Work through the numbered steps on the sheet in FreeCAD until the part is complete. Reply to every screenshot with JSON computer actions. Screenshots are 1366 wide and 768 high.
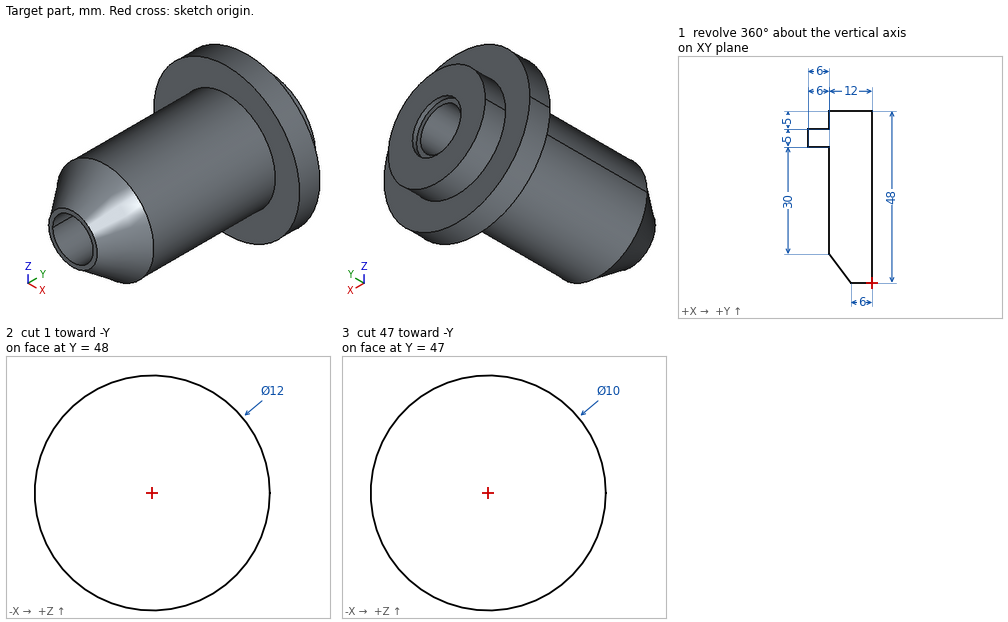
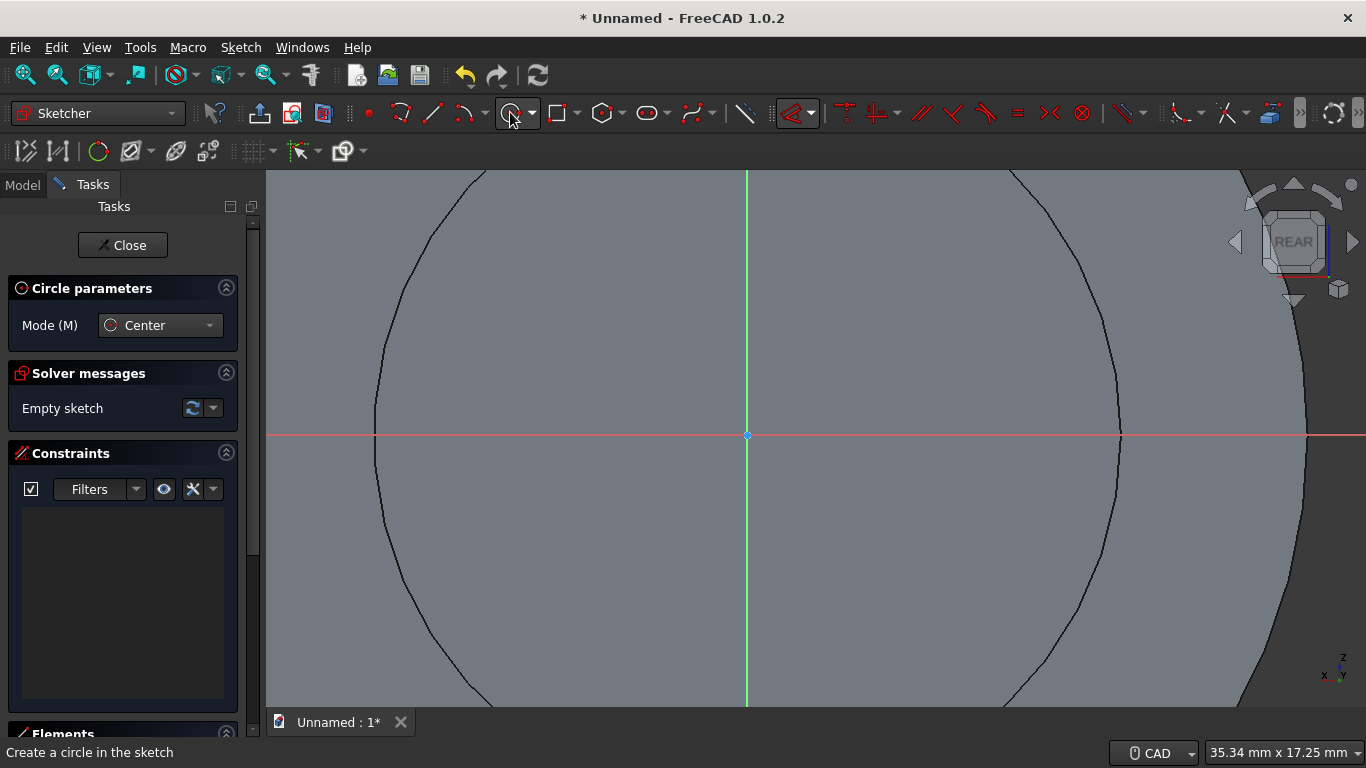
{"action": "left_click", "coordinate": [747, 435]}
{"action": "left_click", "coordinate": [879, 303]}
{"action": "key", "text": "Escape"}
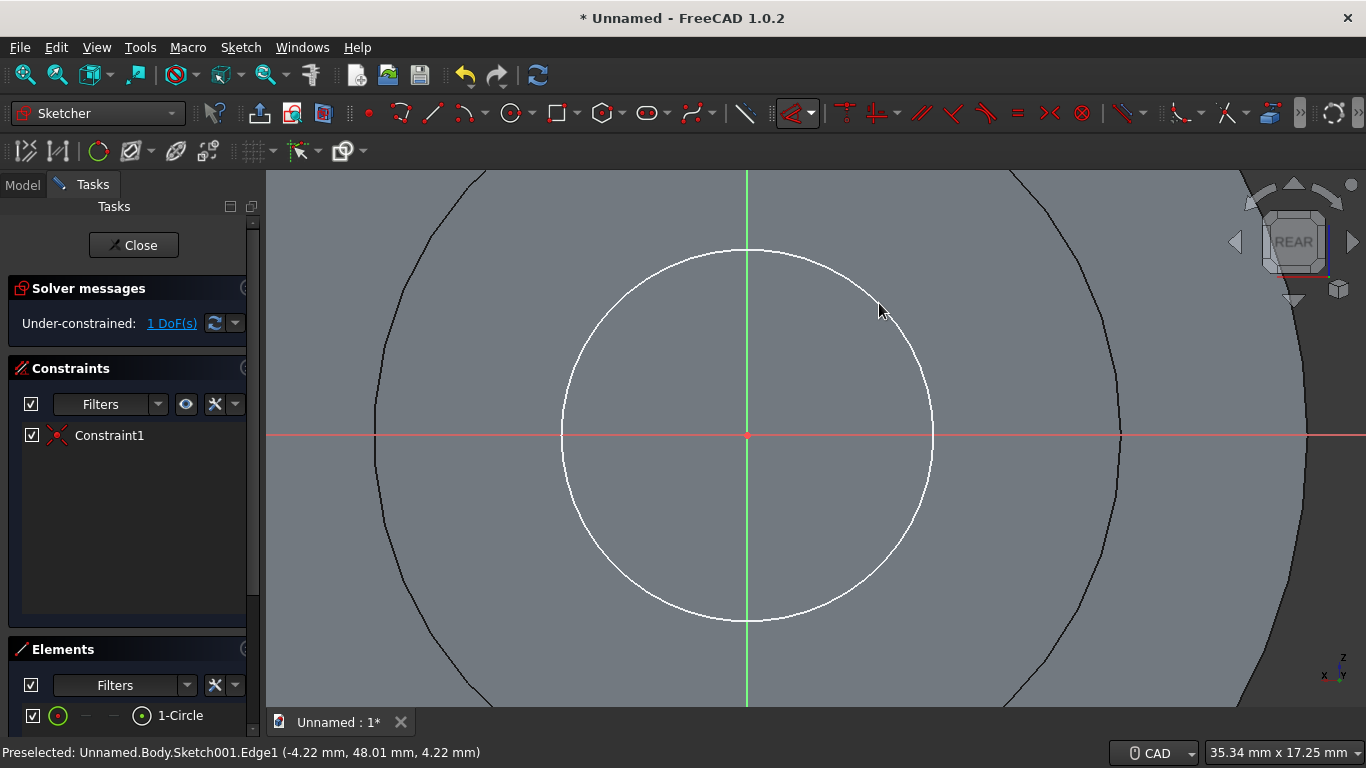
{"action": "left_click", "coordinate": [879, 304]}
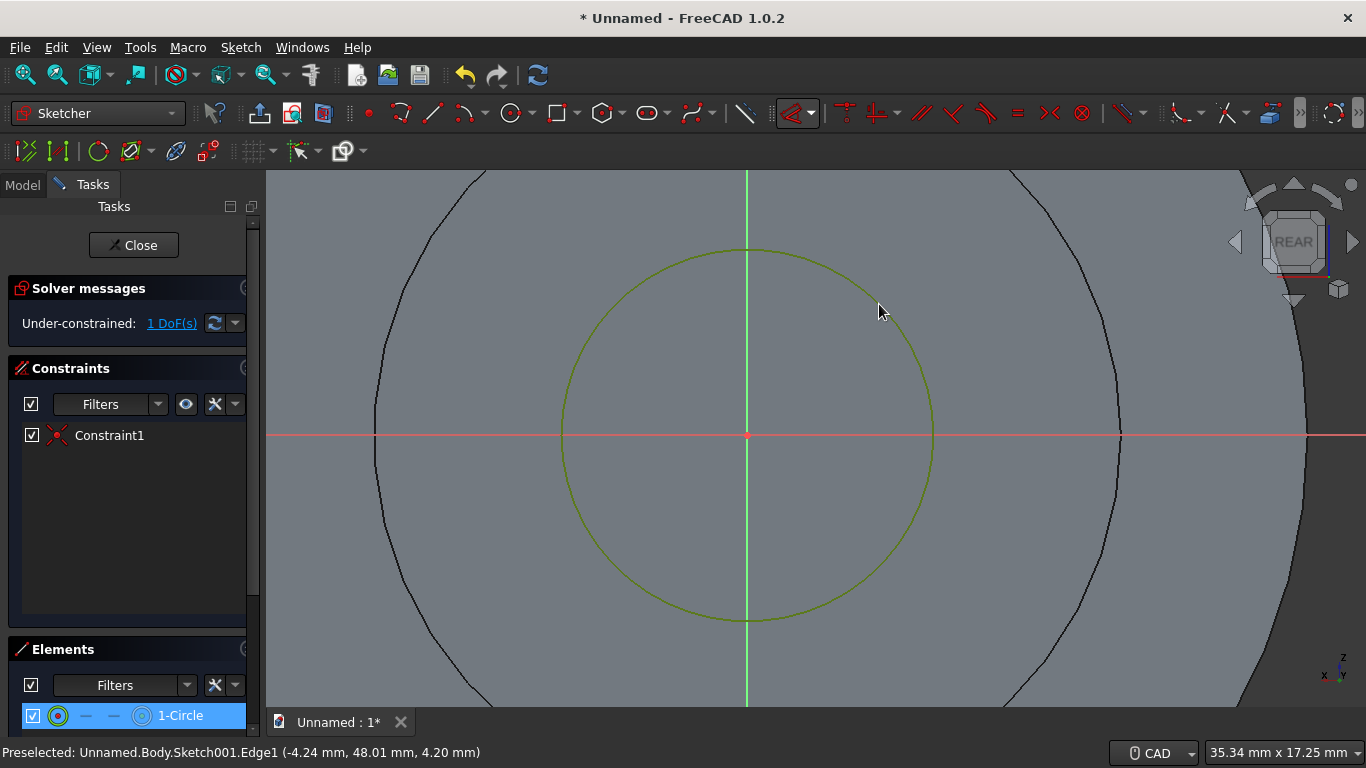
{"action": "left_click", "coordinate": [814, 114]}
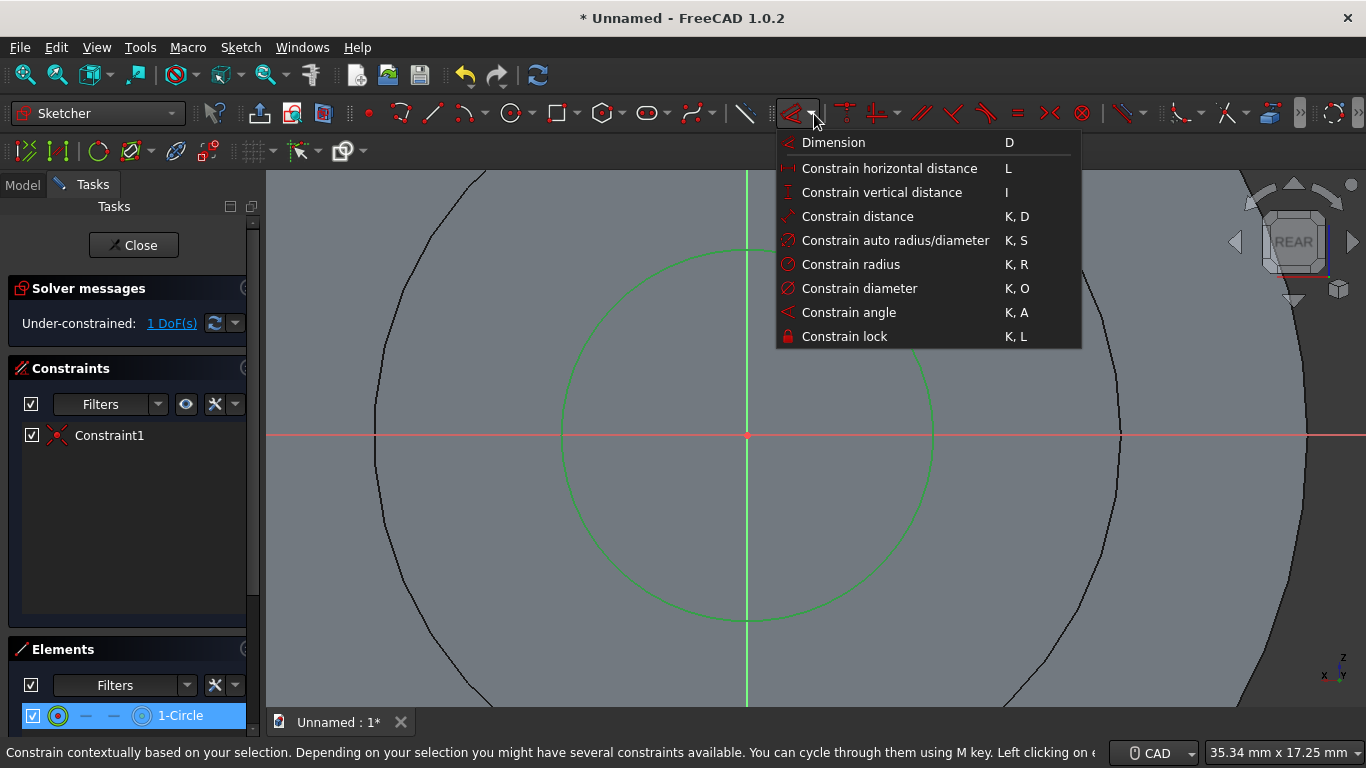
{"action": "left_click", "coordinate": [929, 288]}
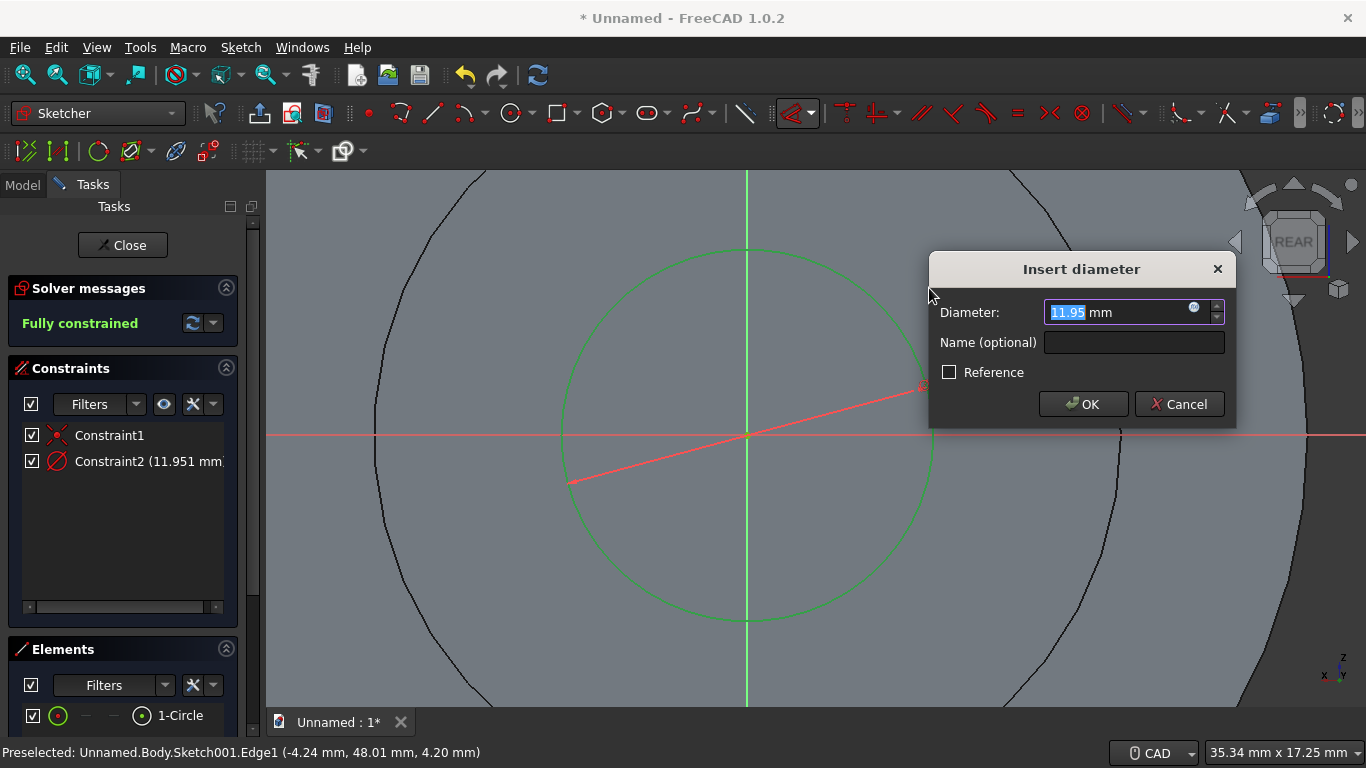
{"action": "type", "text": "12"}
{"action": "key", "text": "Return"}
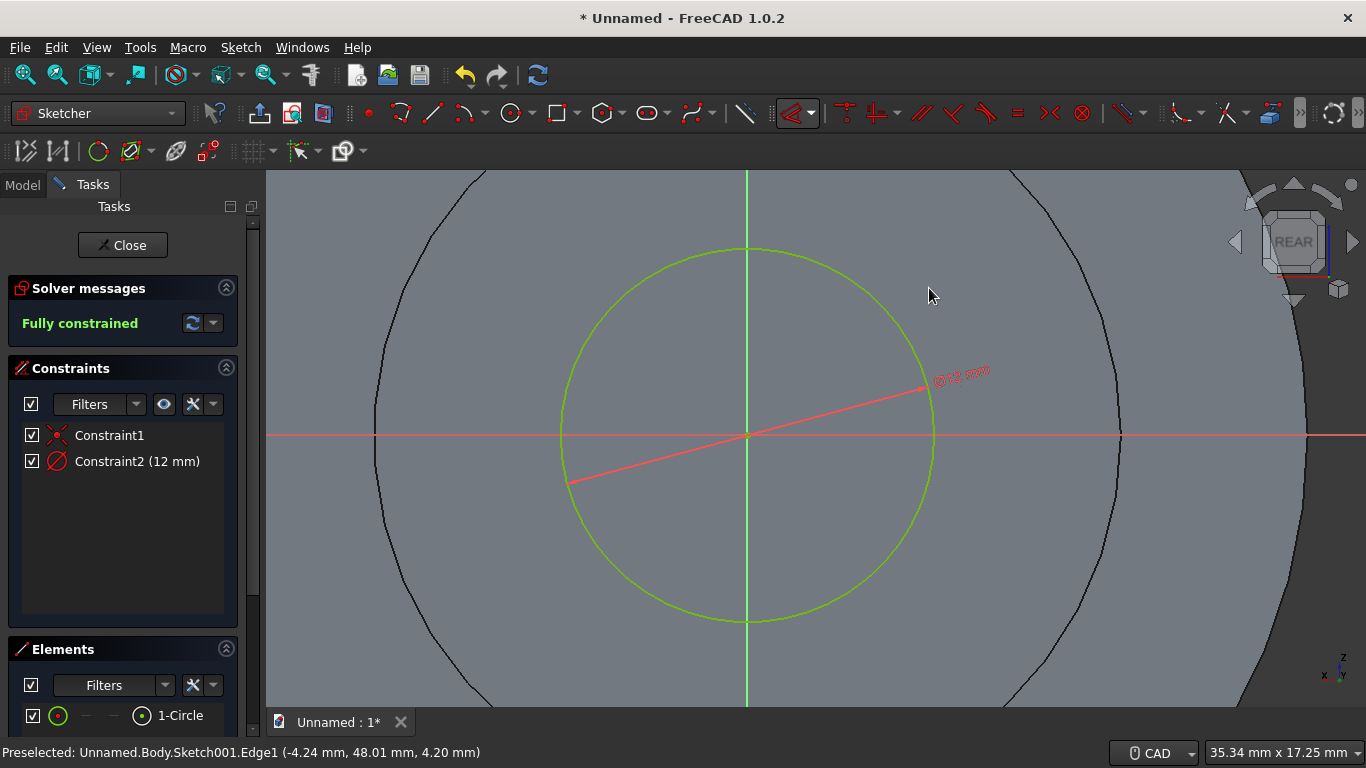
{"action": "left_click", "coordinate": [123, 245]}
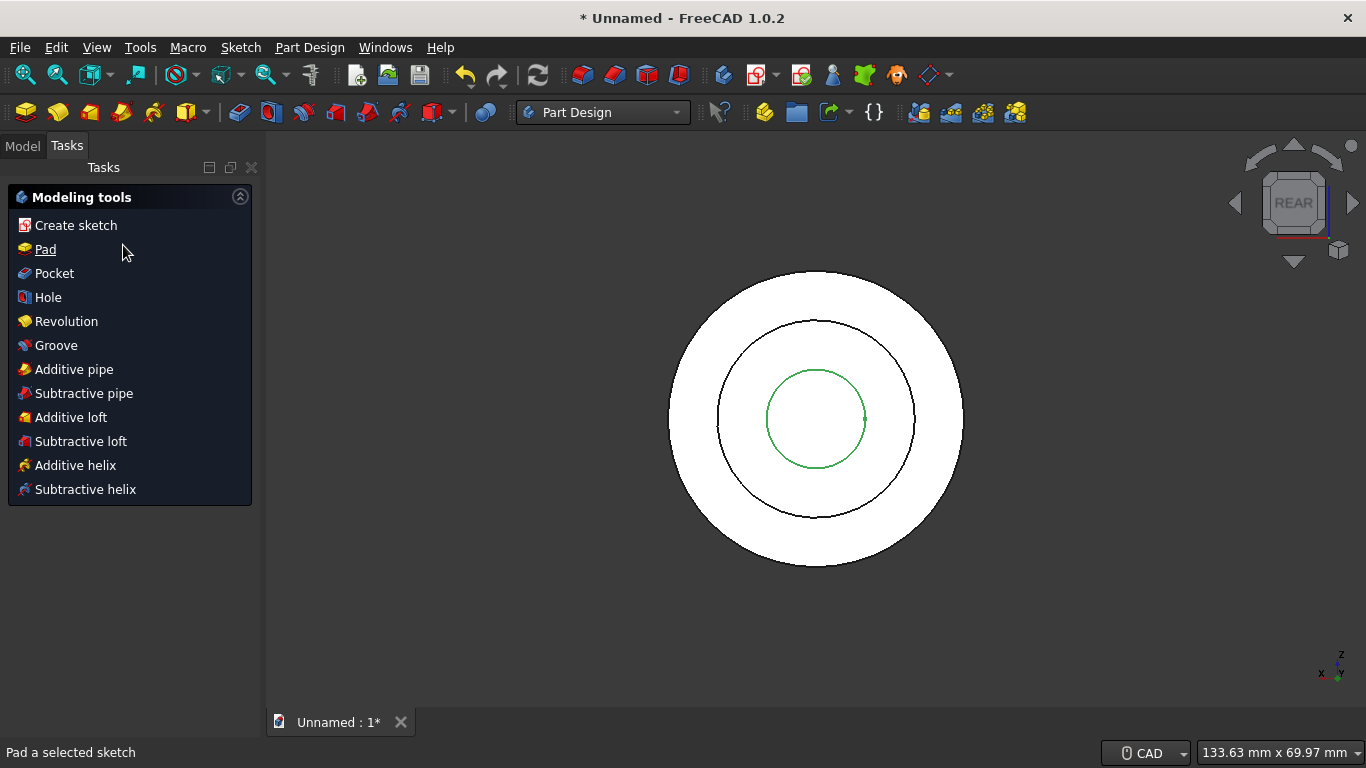
{"action": "left_click", "coordinate": [240, 112]}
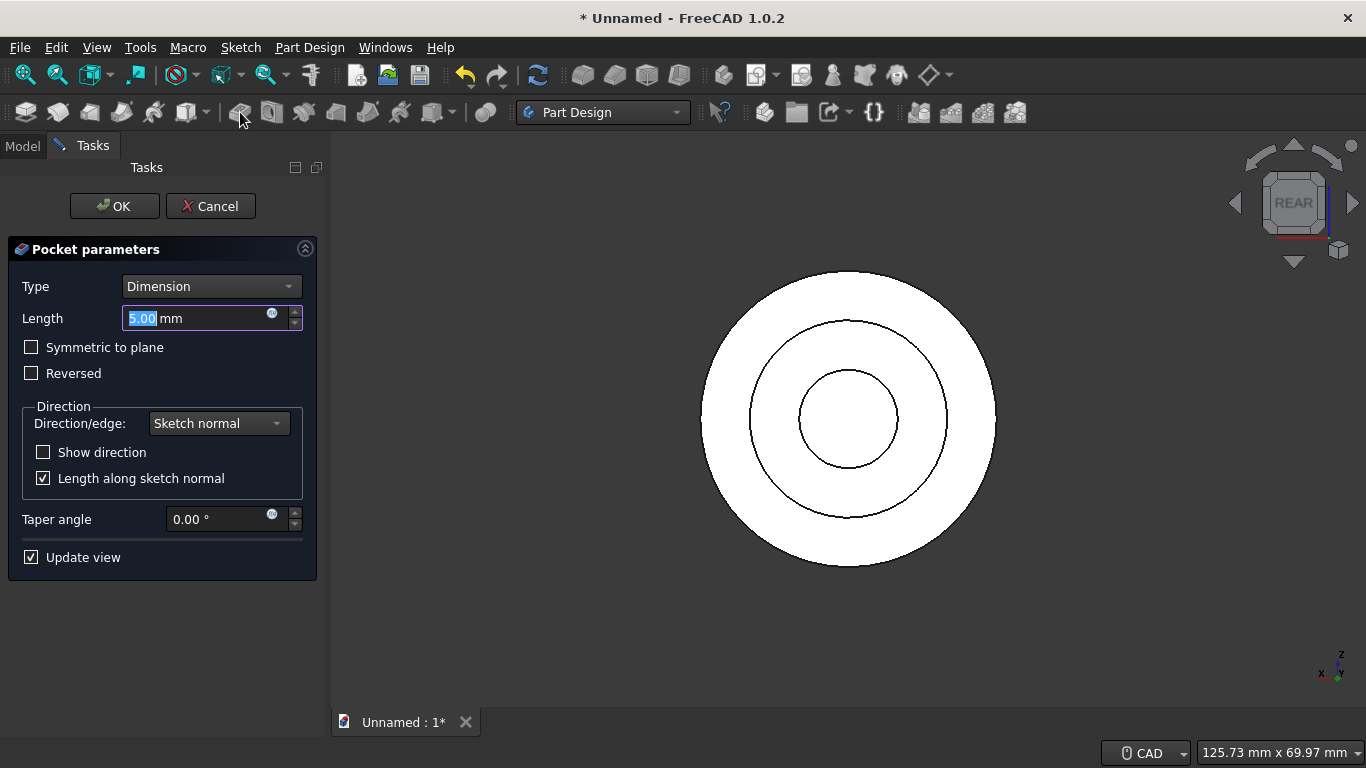
{"action": "type", "text": "1"}
{"action": "key", "text": "Tab"}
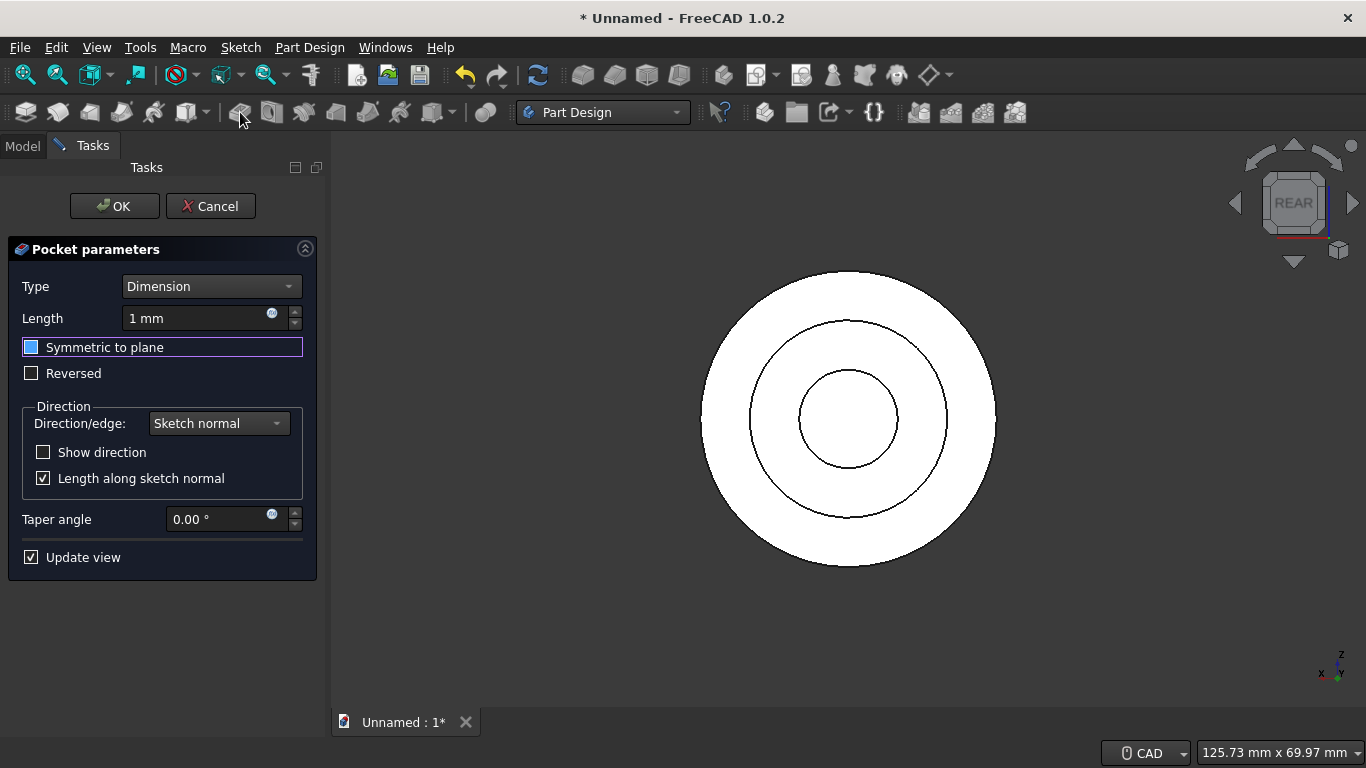
{"action": "left_click", "coordinate": [115, 206]}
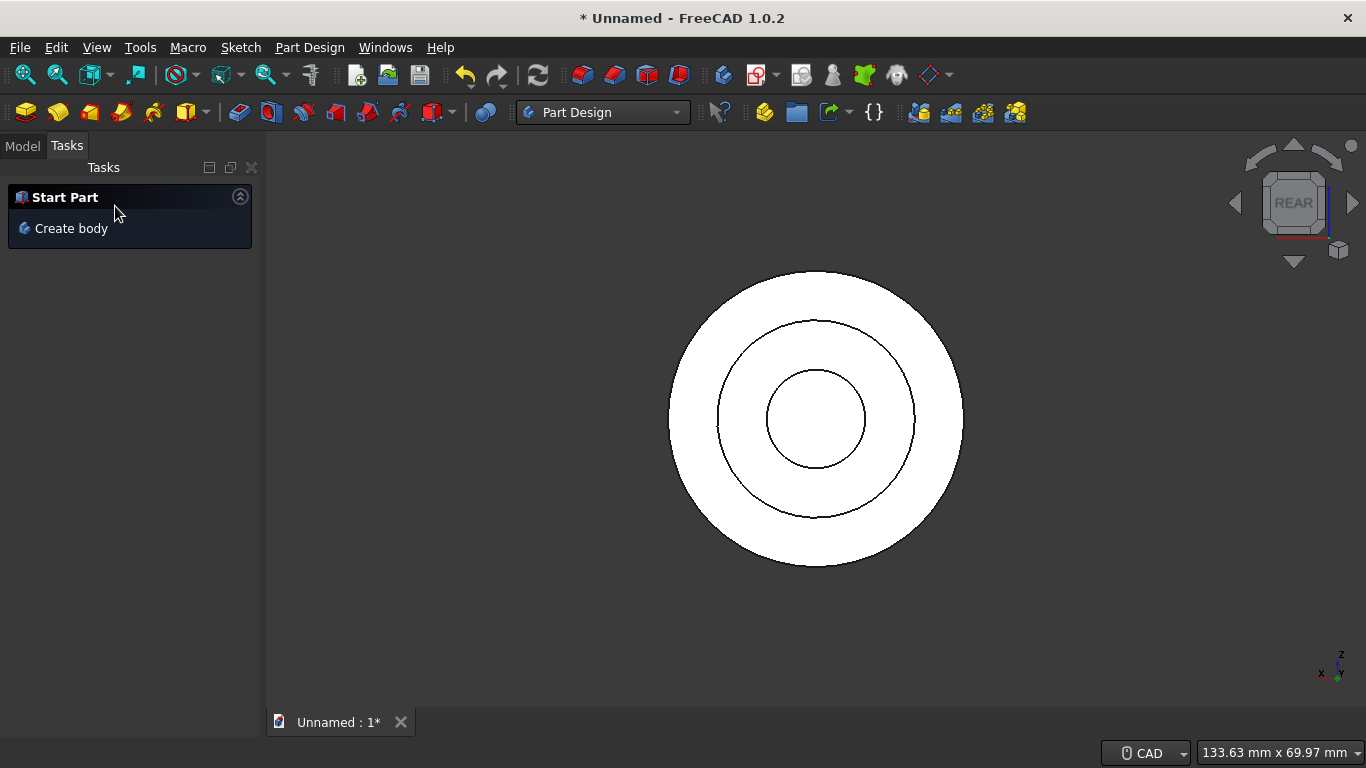
{"action": "left_click", "coordinate": [816, 418]}